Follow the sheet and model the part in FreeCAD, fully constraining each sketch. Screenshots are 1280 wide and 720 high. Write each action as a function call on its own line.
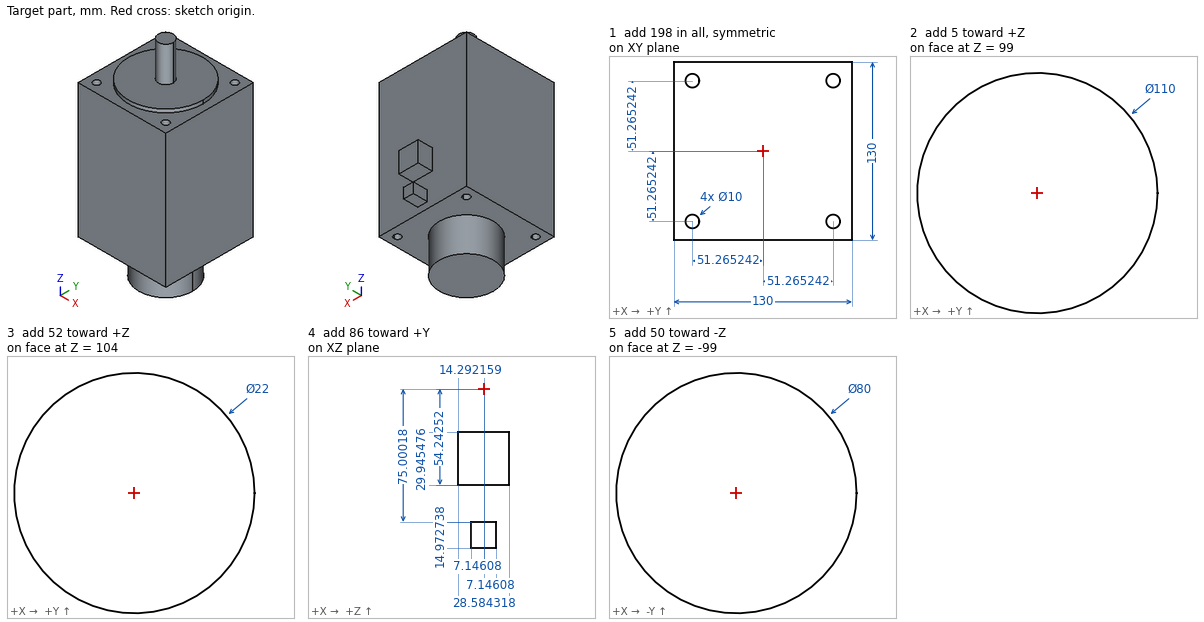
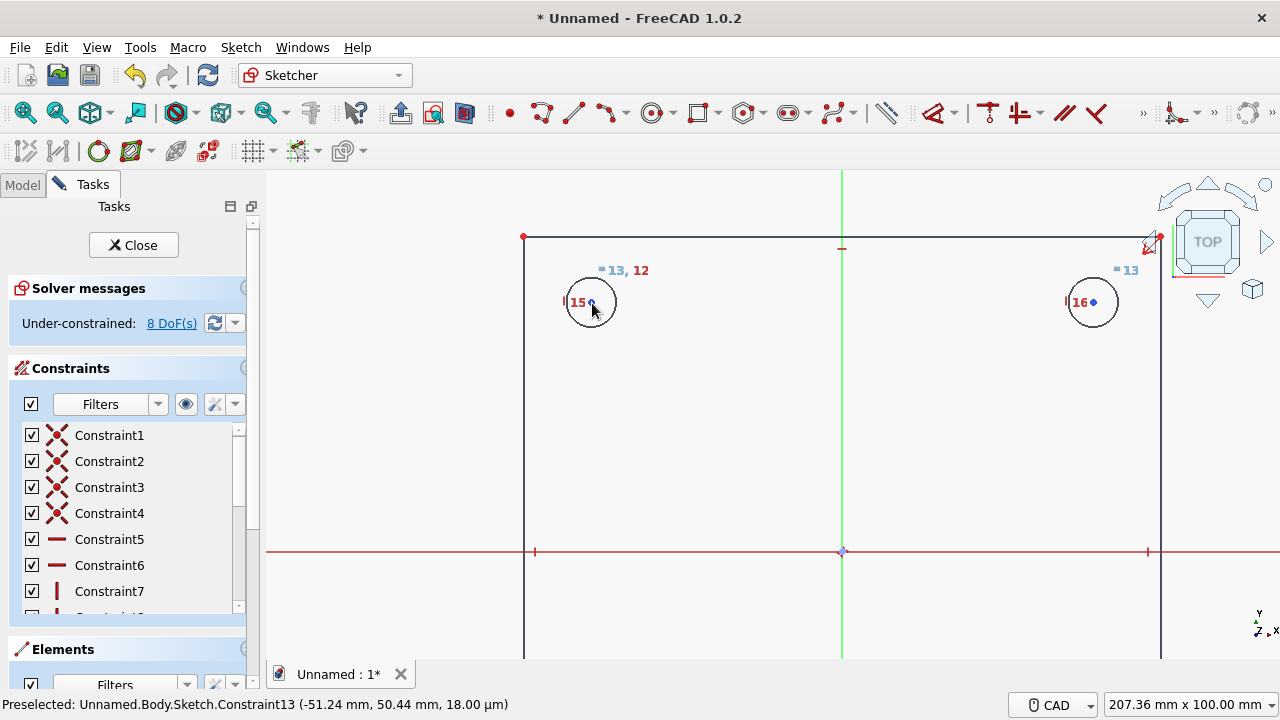
click(591, 302)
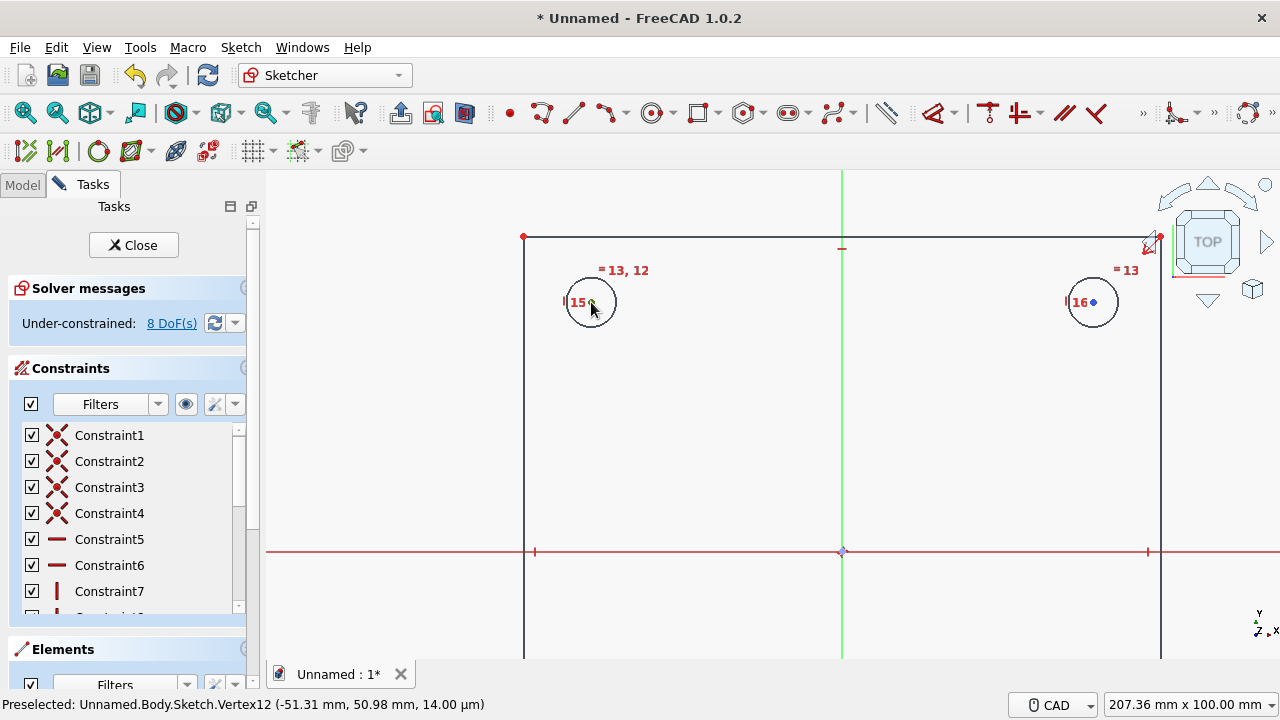
click(1093, 302)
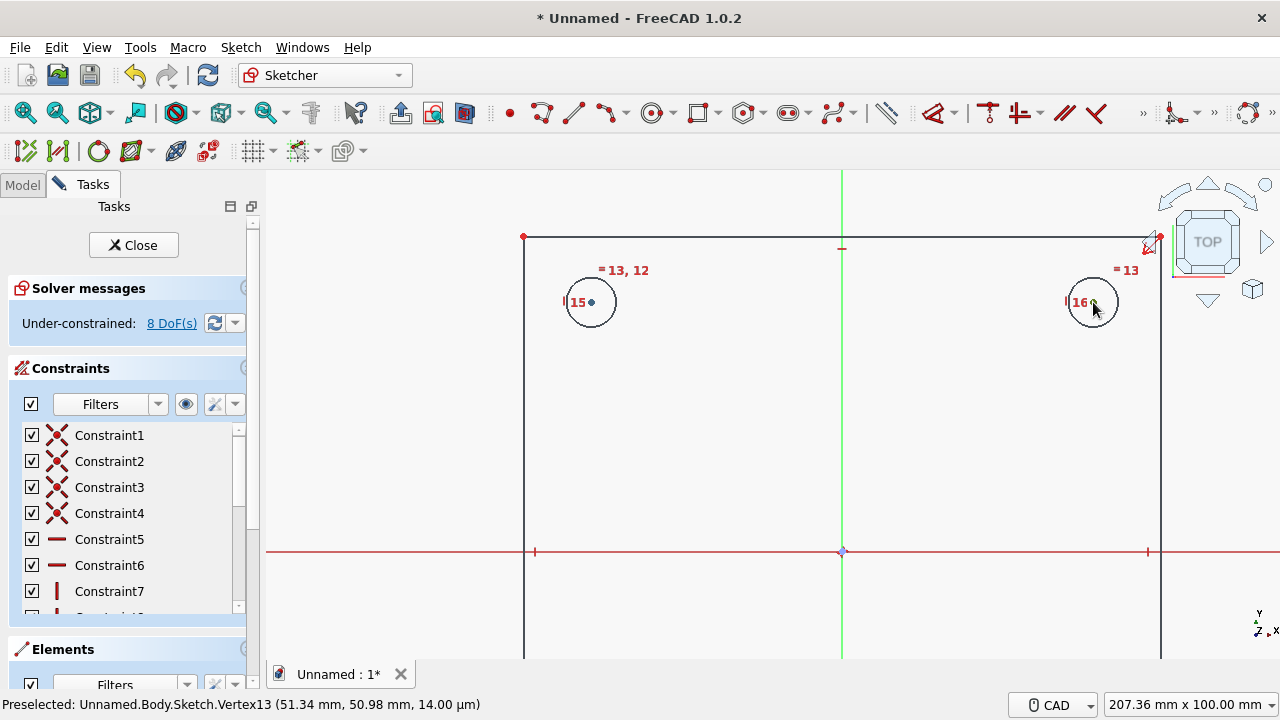
key(h)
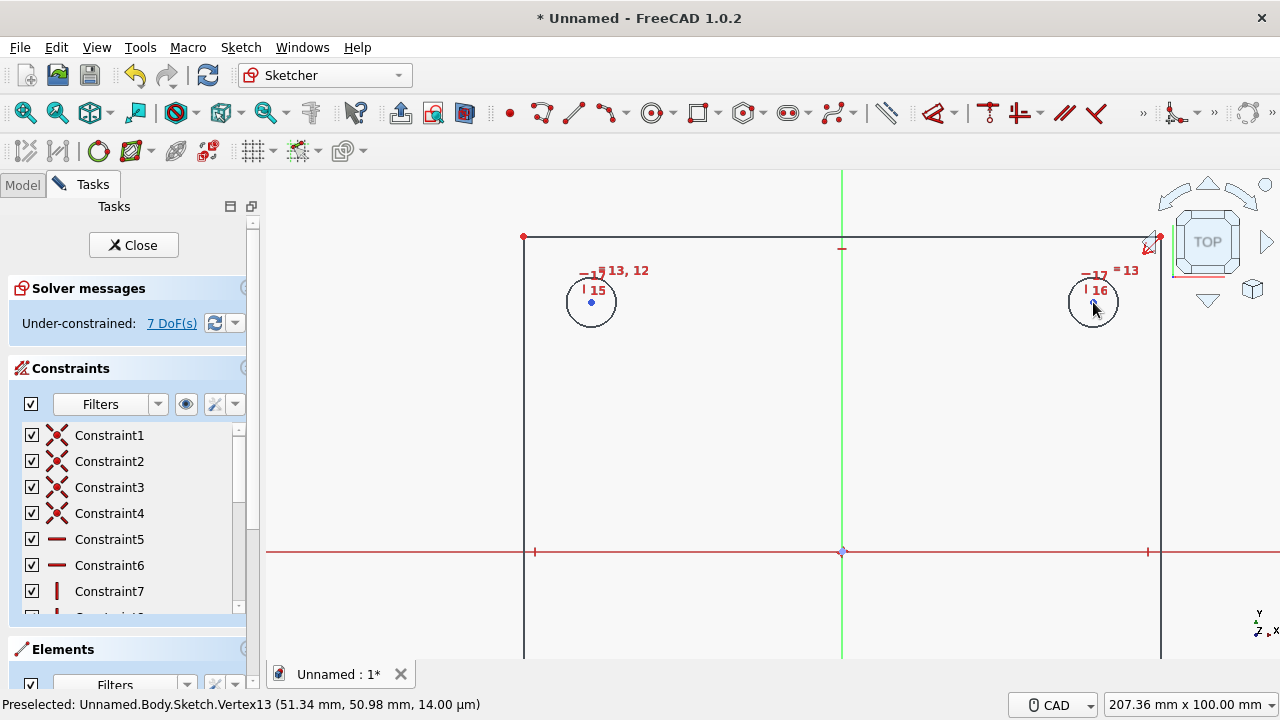
key(d)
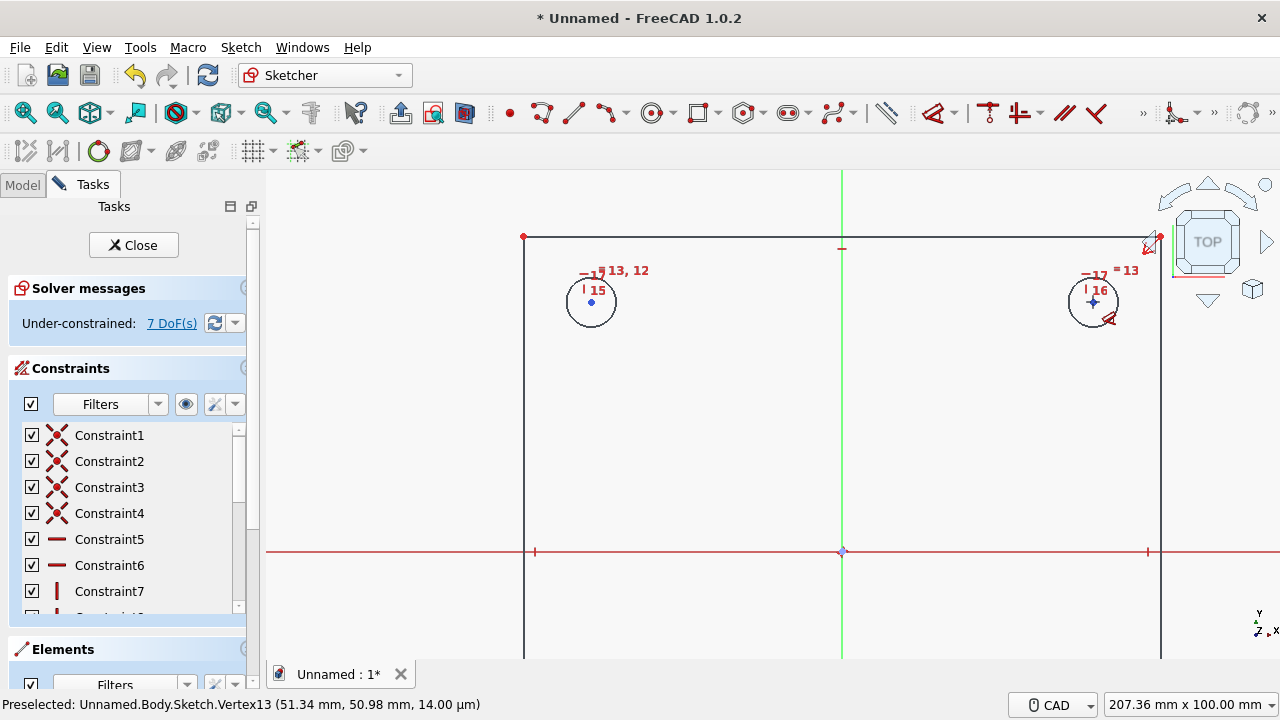
scroll(592, 303, down, 4)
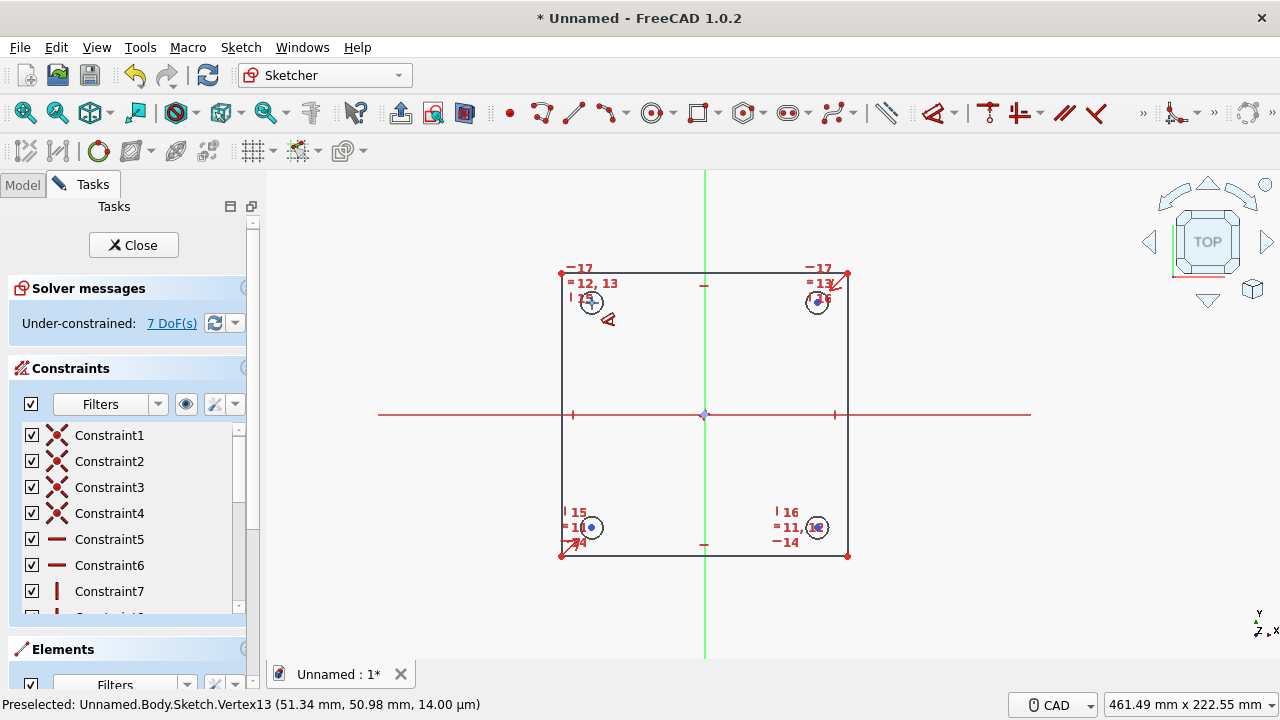
scroll(600, 520, up, 3)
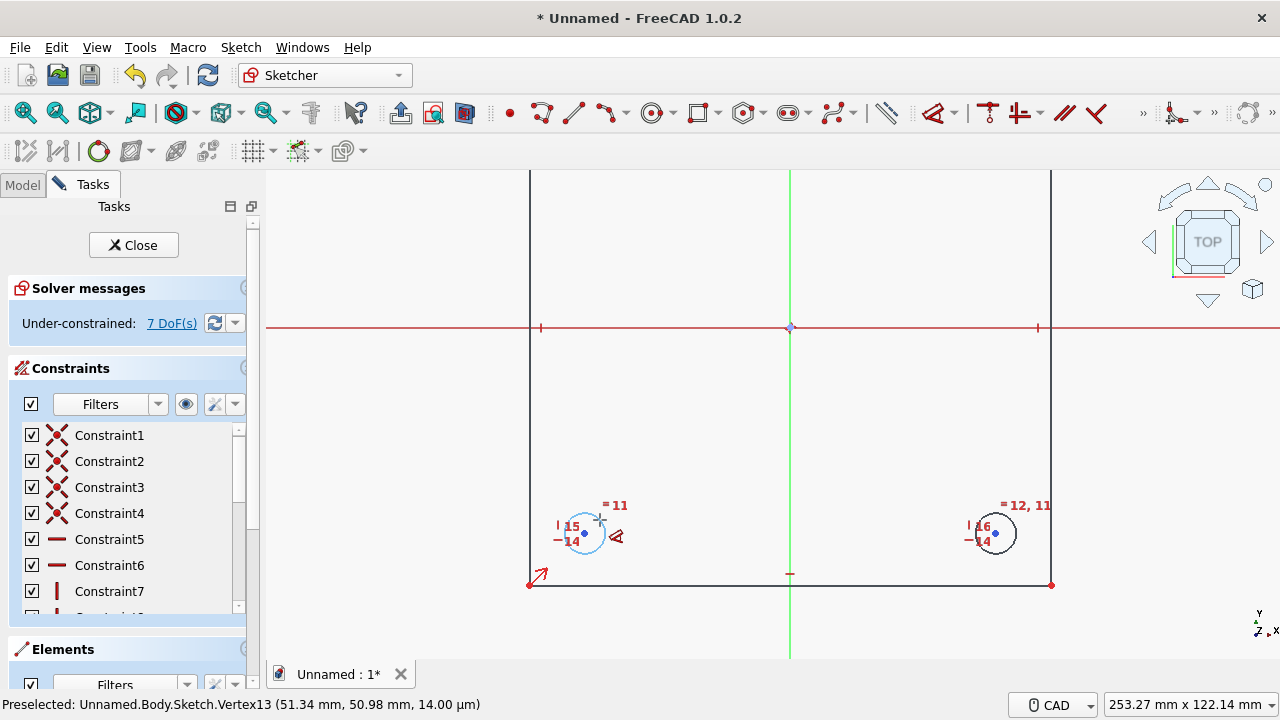
click(599, 519)
click(621, 496)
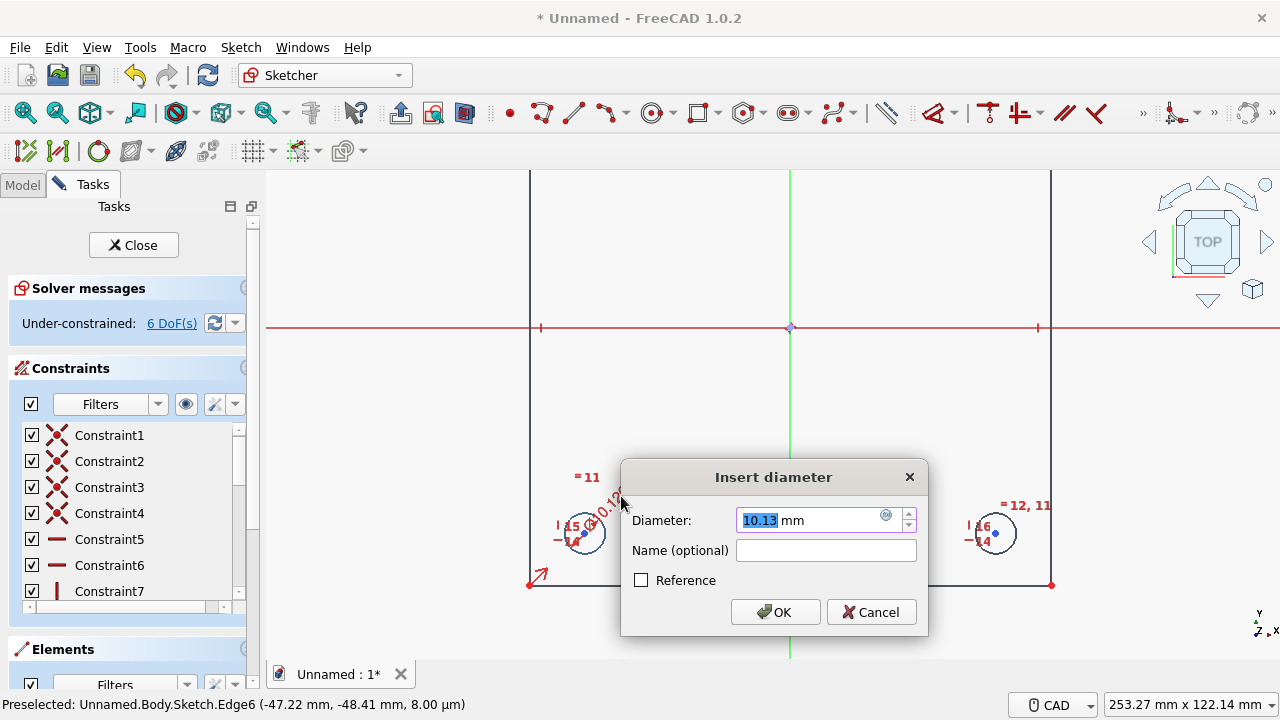
text(10)
key(Return)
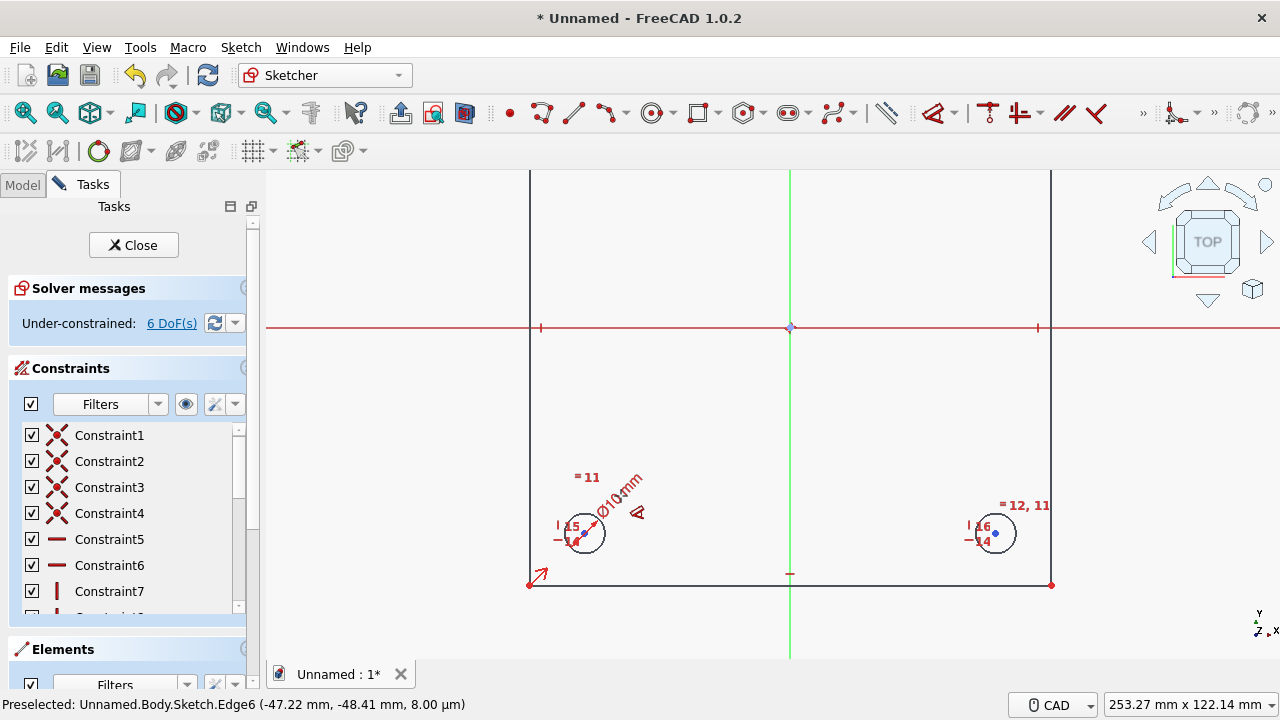
click(686, 586)
click(670, 620)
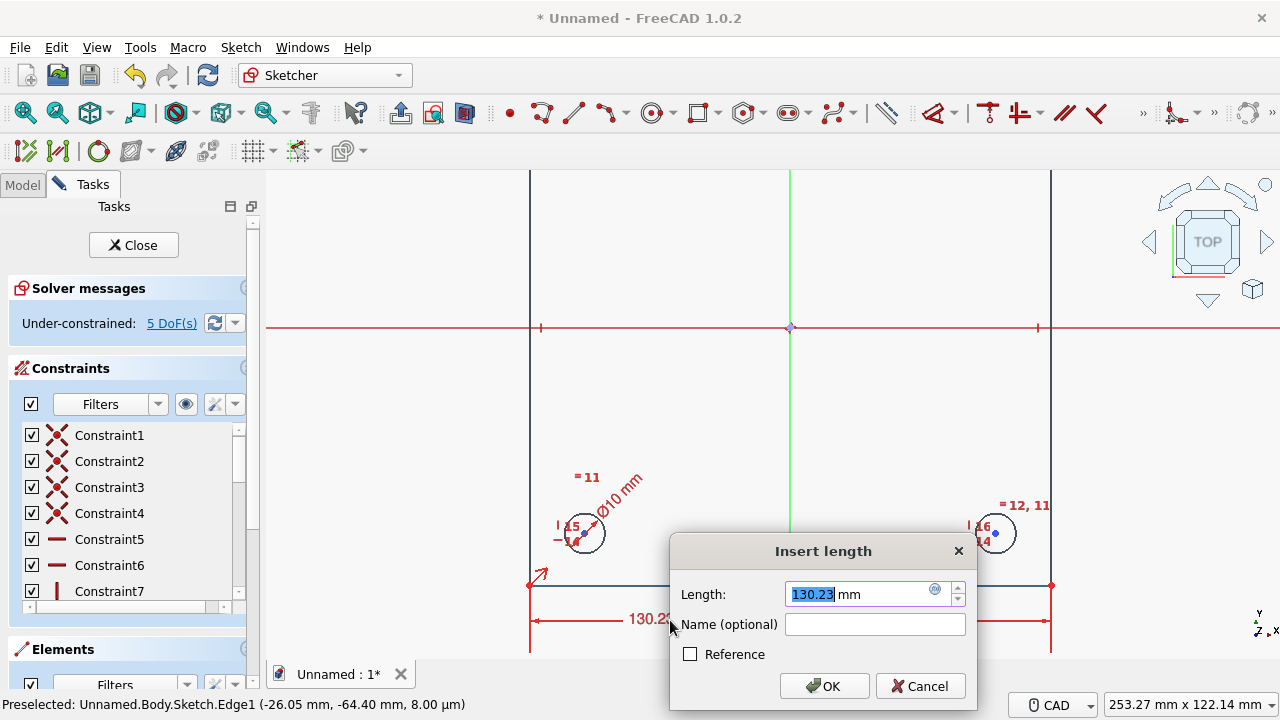
text(130)
key(Return)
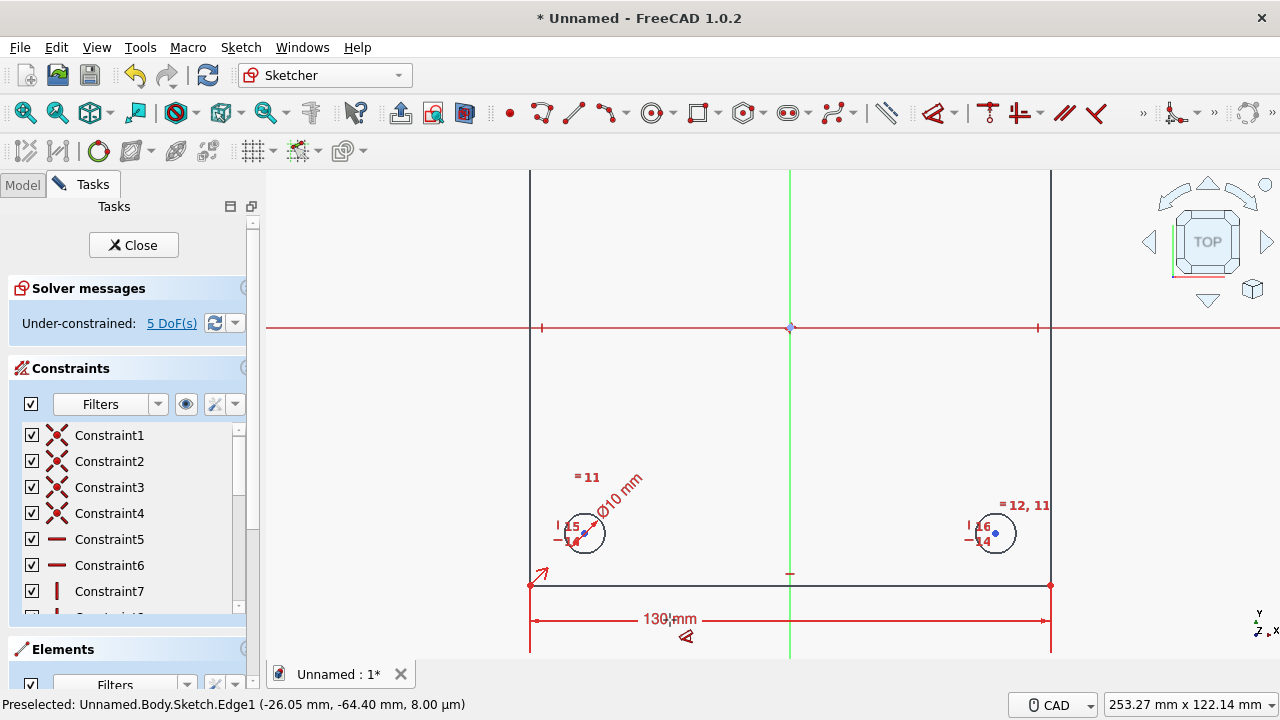
click(1051, 431)
click(1085, 392)